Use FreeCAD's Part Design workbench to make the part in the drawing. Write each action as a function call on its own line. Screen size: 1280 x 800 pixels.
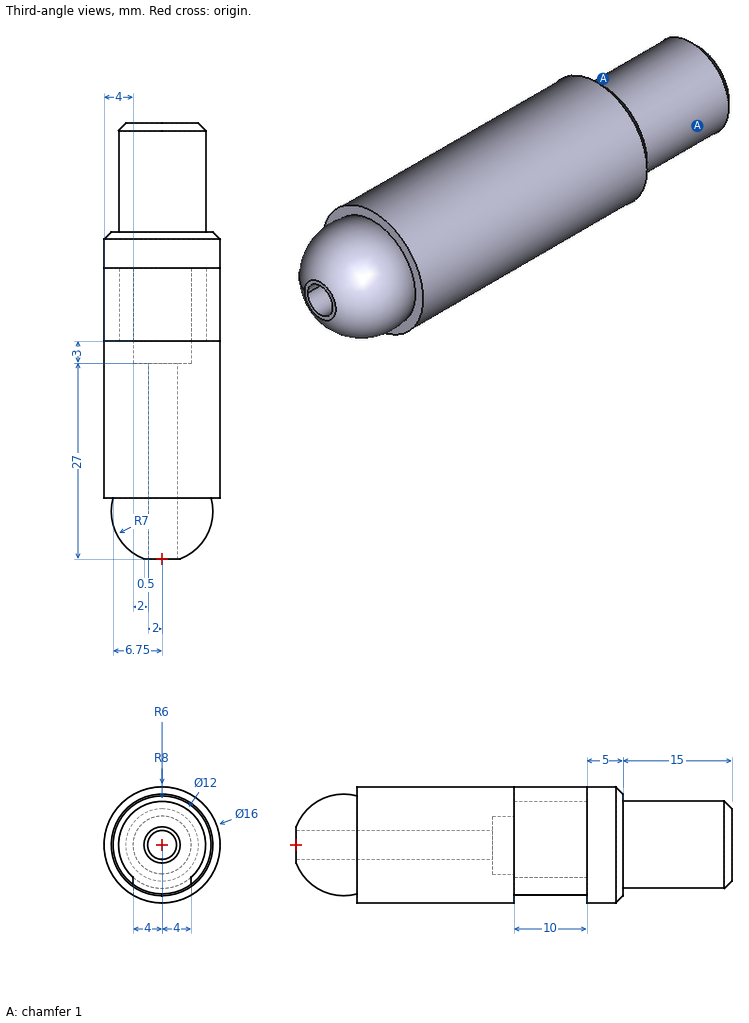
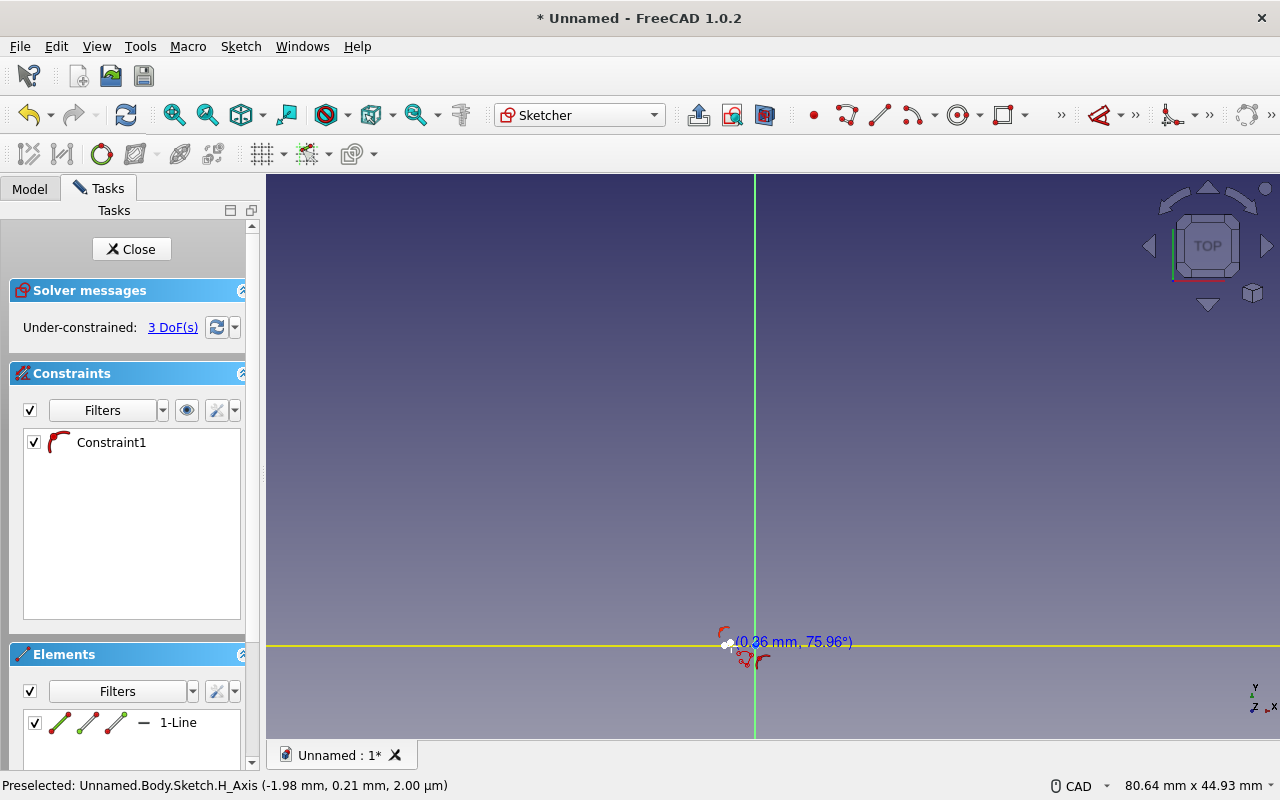
click(730, 306)
click(705, 306)
click(705, 268)
click(655, 268)
click(655, 540)
click(670, 540)
right_click(670, 540)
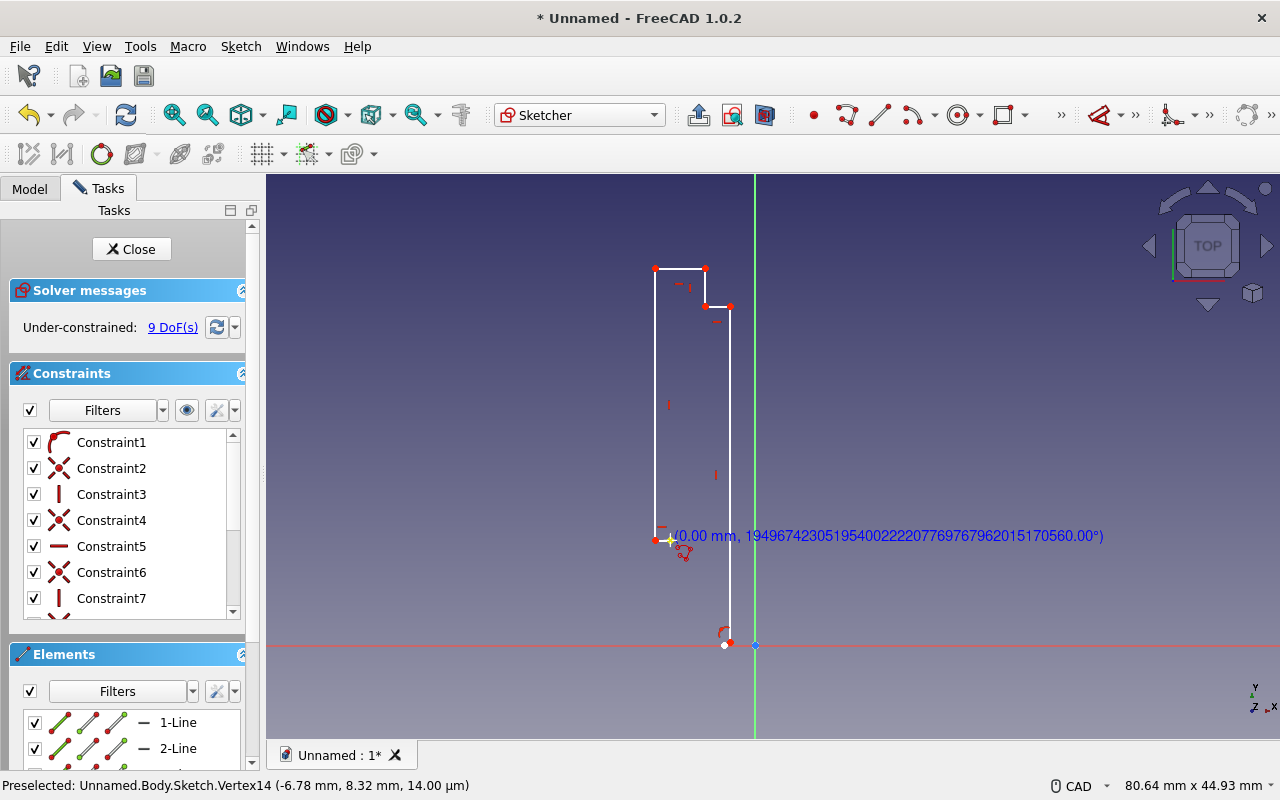
click(934, 116)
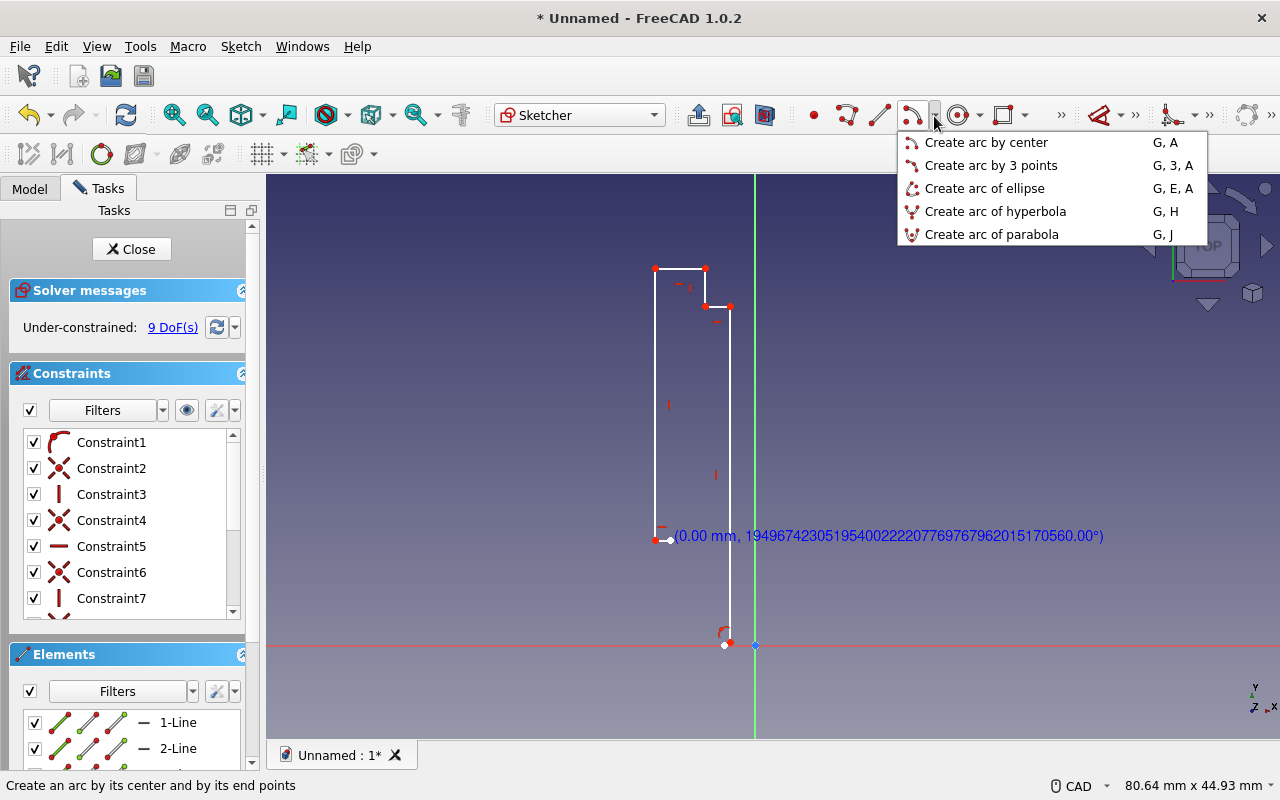
click(1052, 166)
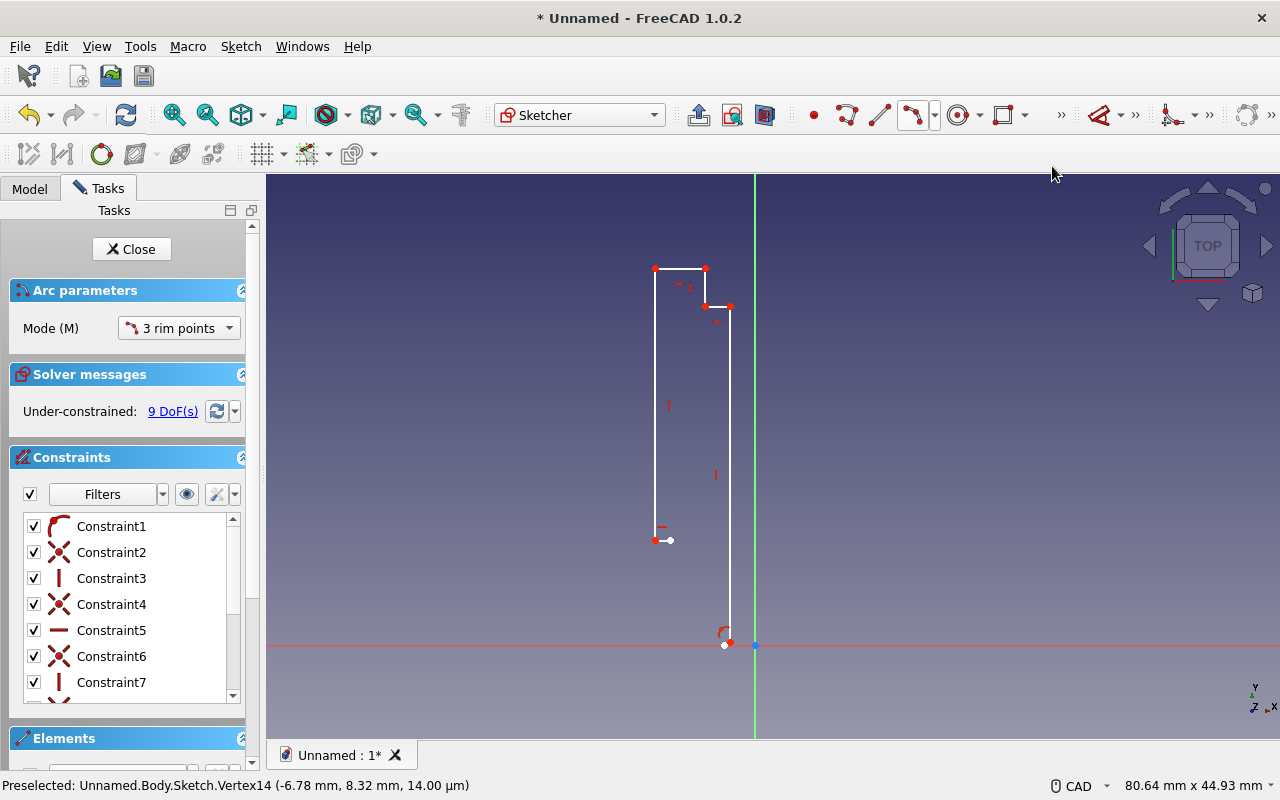
scroll(670, 540, up, 4)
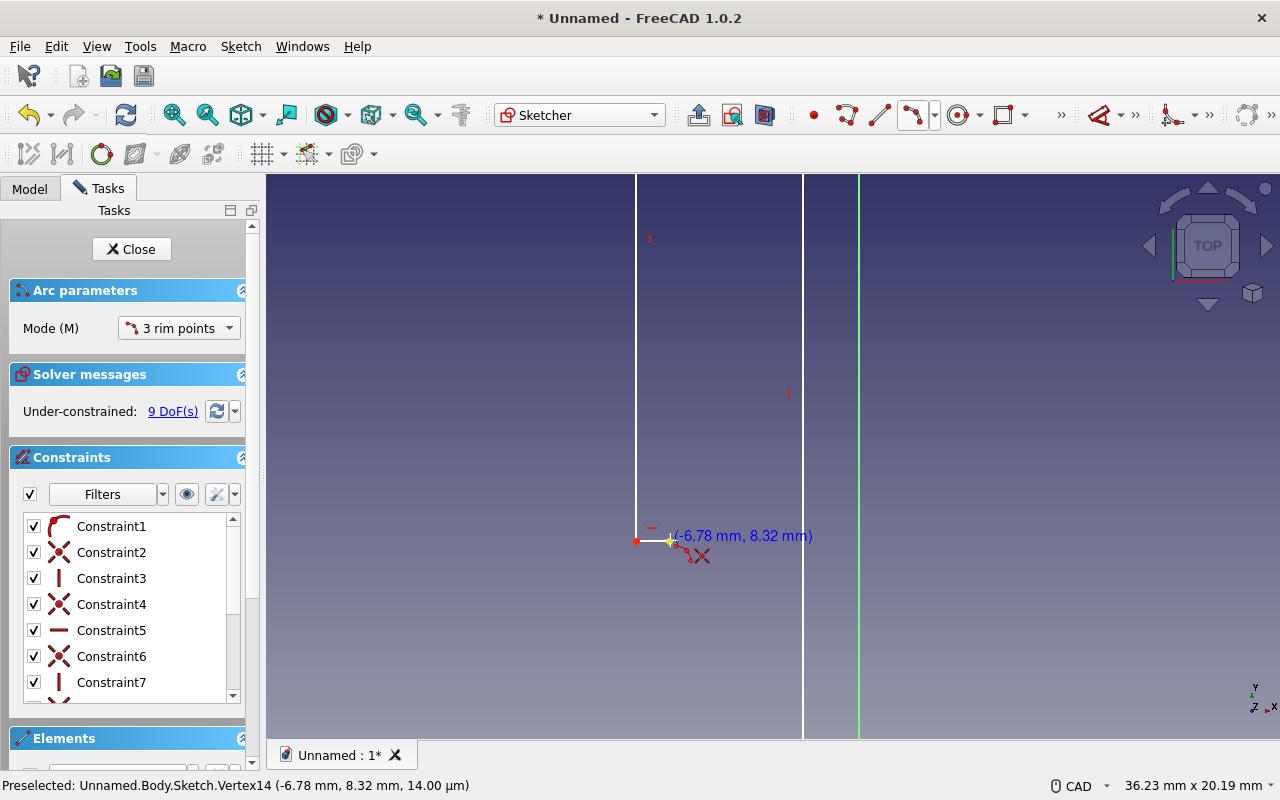
click(670, 541)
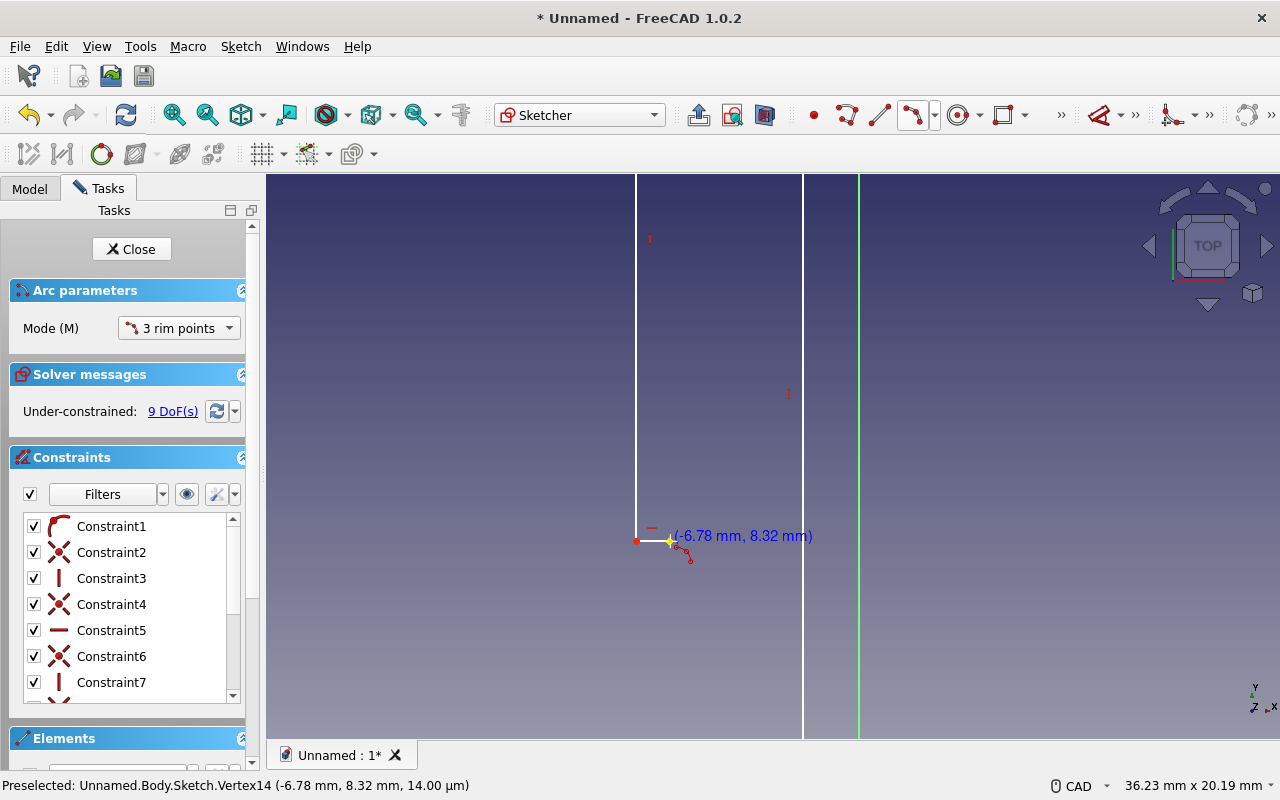
scroll(670, 540, down, 4)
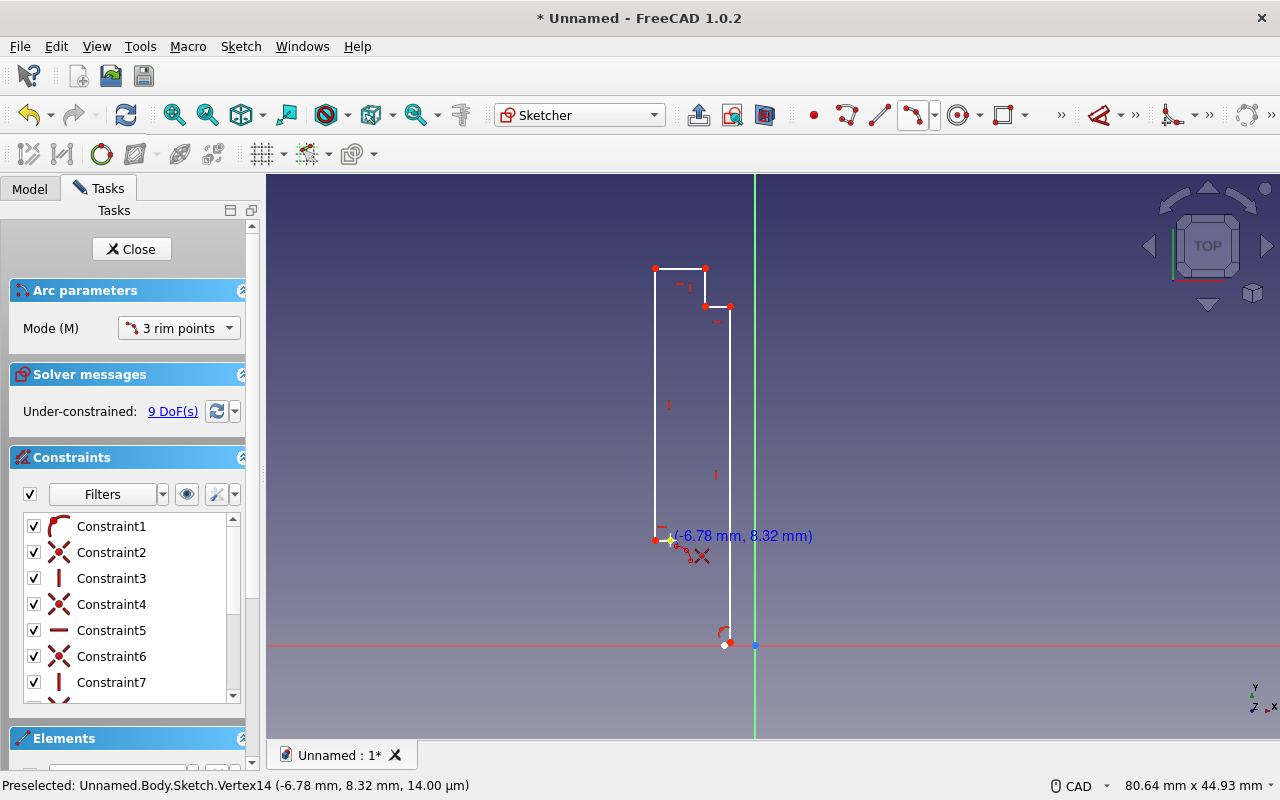
scroll(724, 646, up, 9)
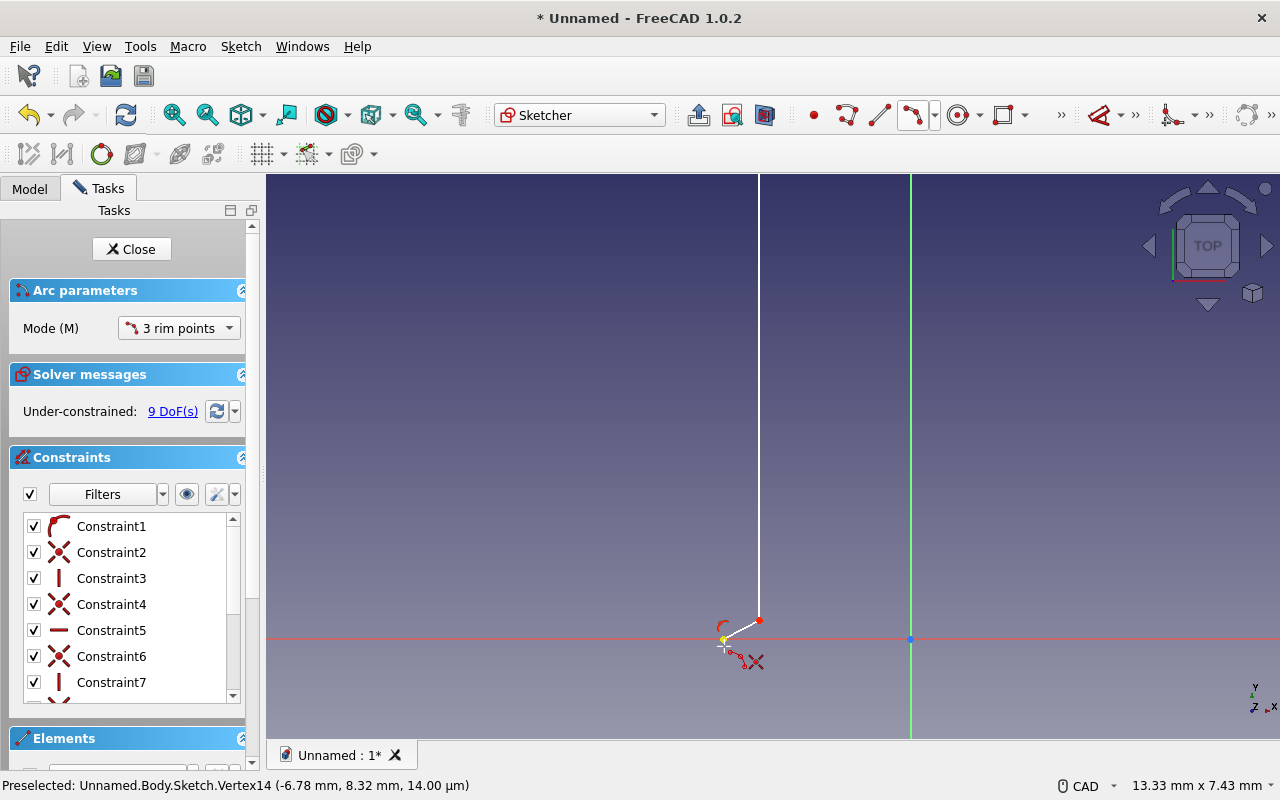
click(723, 639)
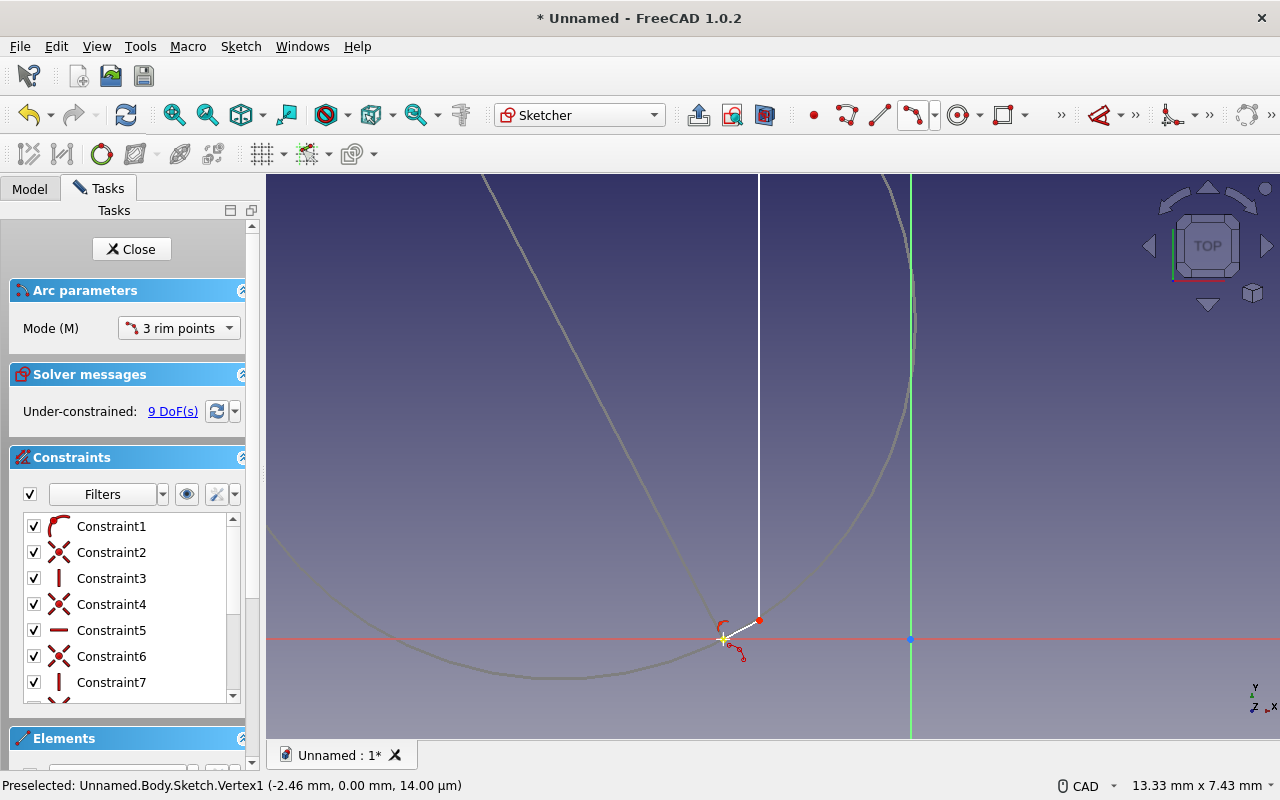
scroll(724, 646, down, 9)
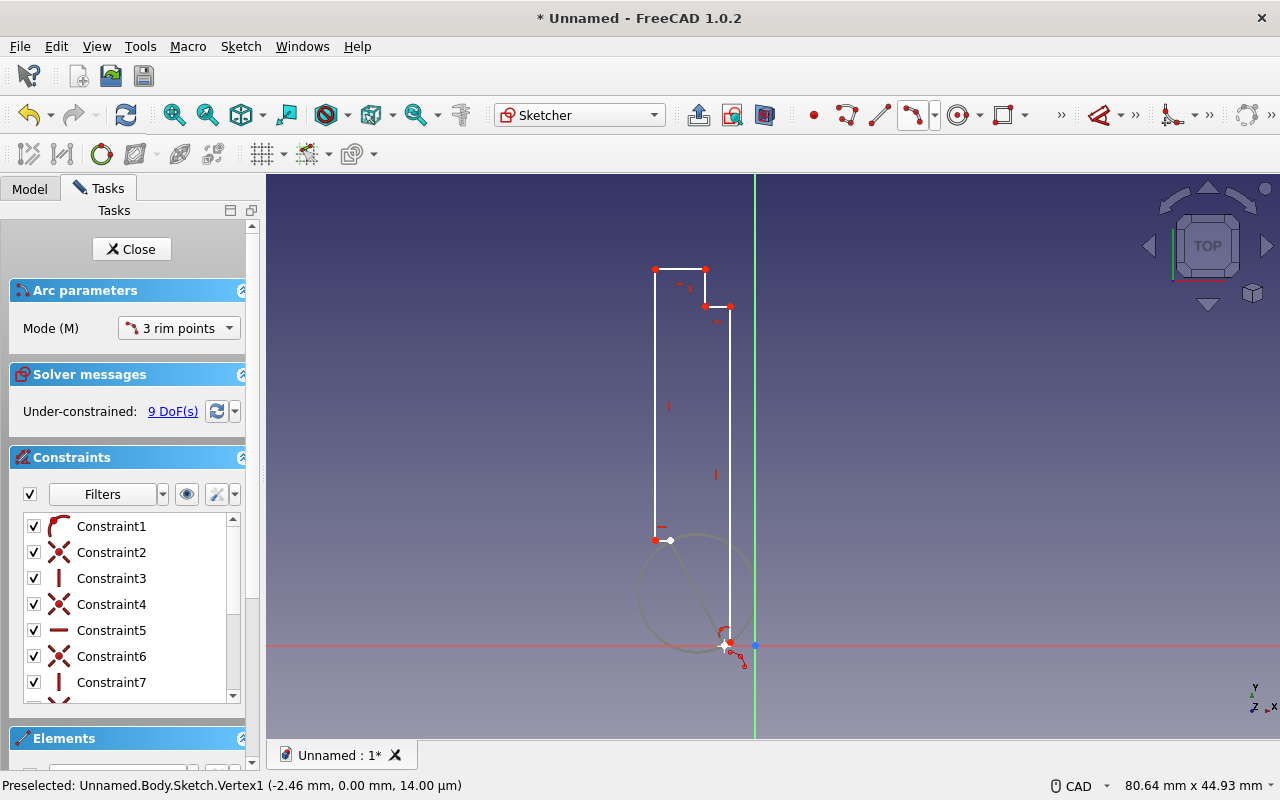
click(677, 603)
key(Escape)